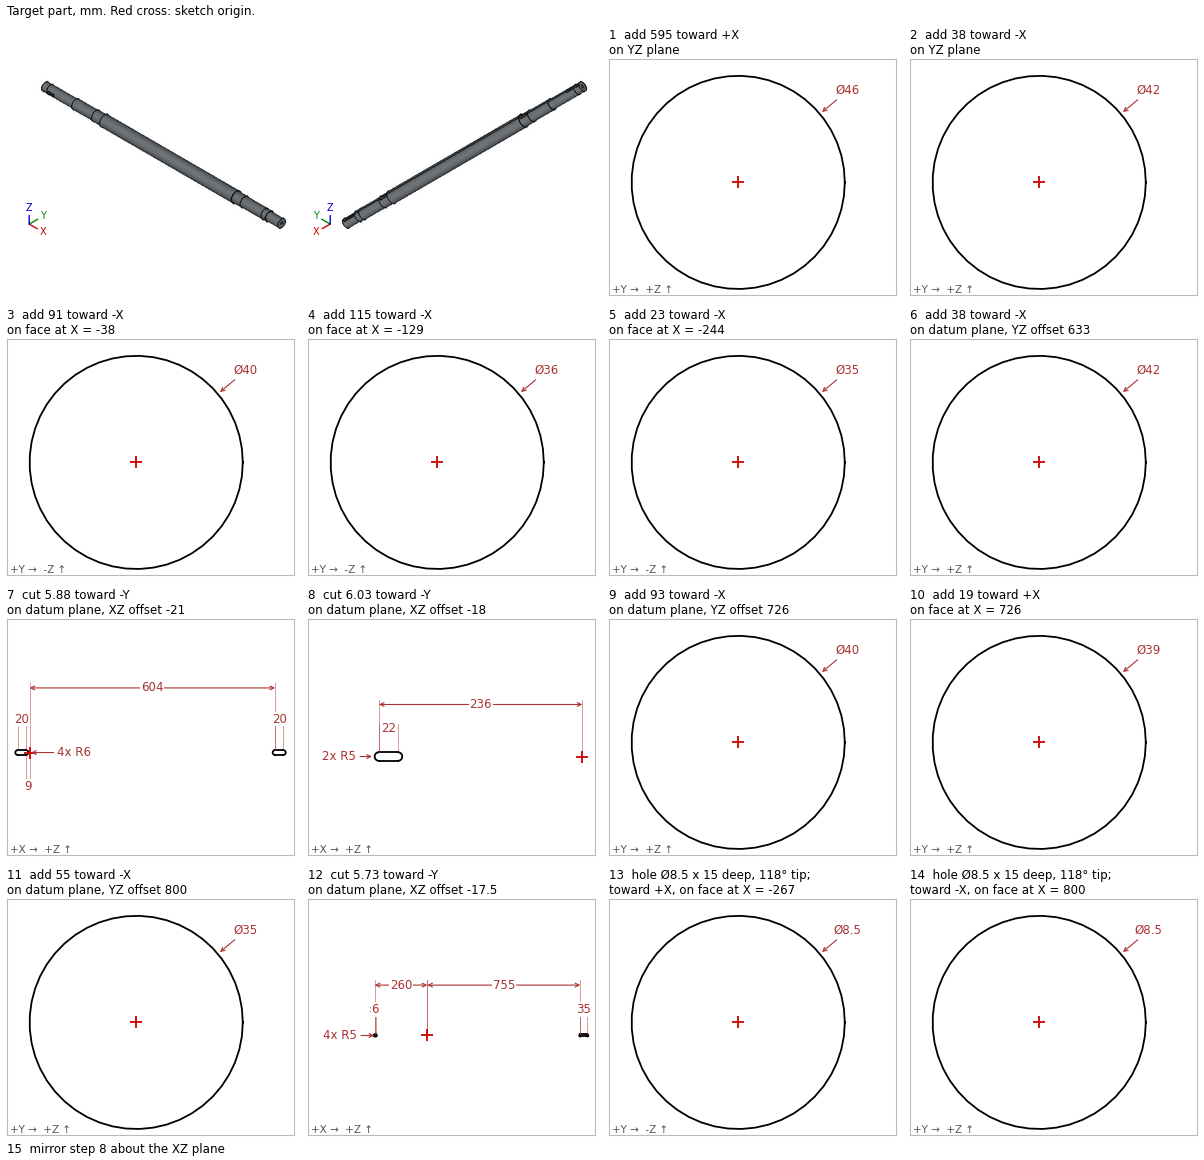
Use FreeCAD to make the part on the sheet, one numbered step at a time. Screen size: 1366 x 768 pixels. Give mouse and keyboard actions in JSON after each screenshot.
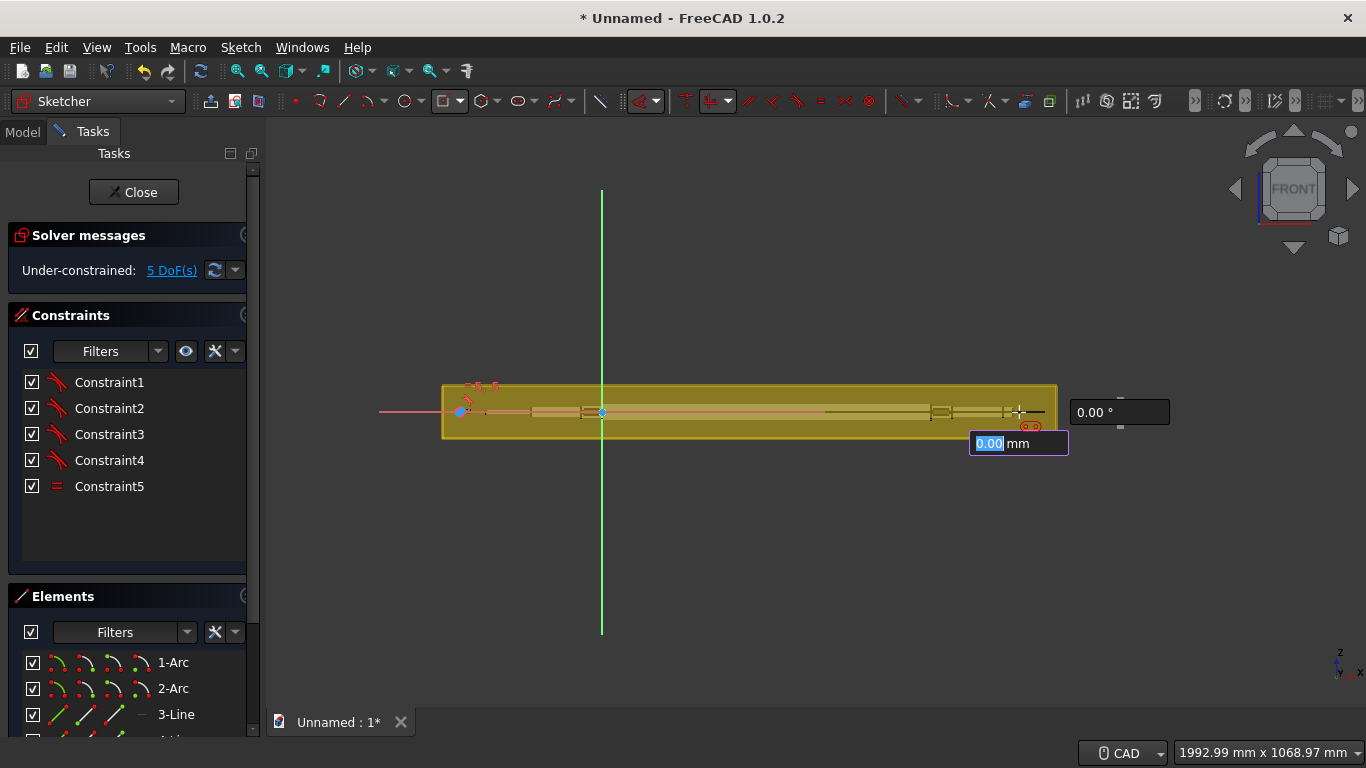
{"action": "left_click", "coordinate": [1038, 403]}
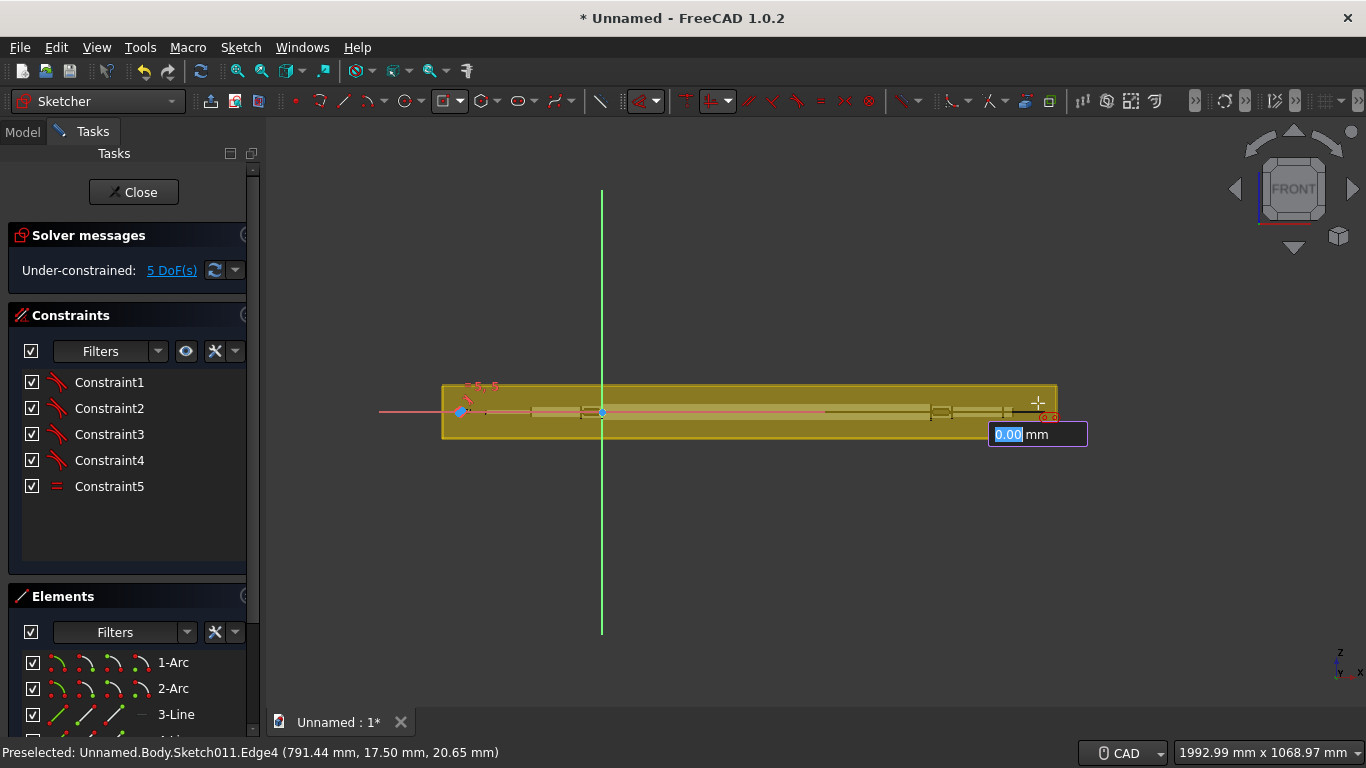
{"action": "scroll", "coordinate": [1029, 409], "scroll_direction": "up", "scroll_amount": 9}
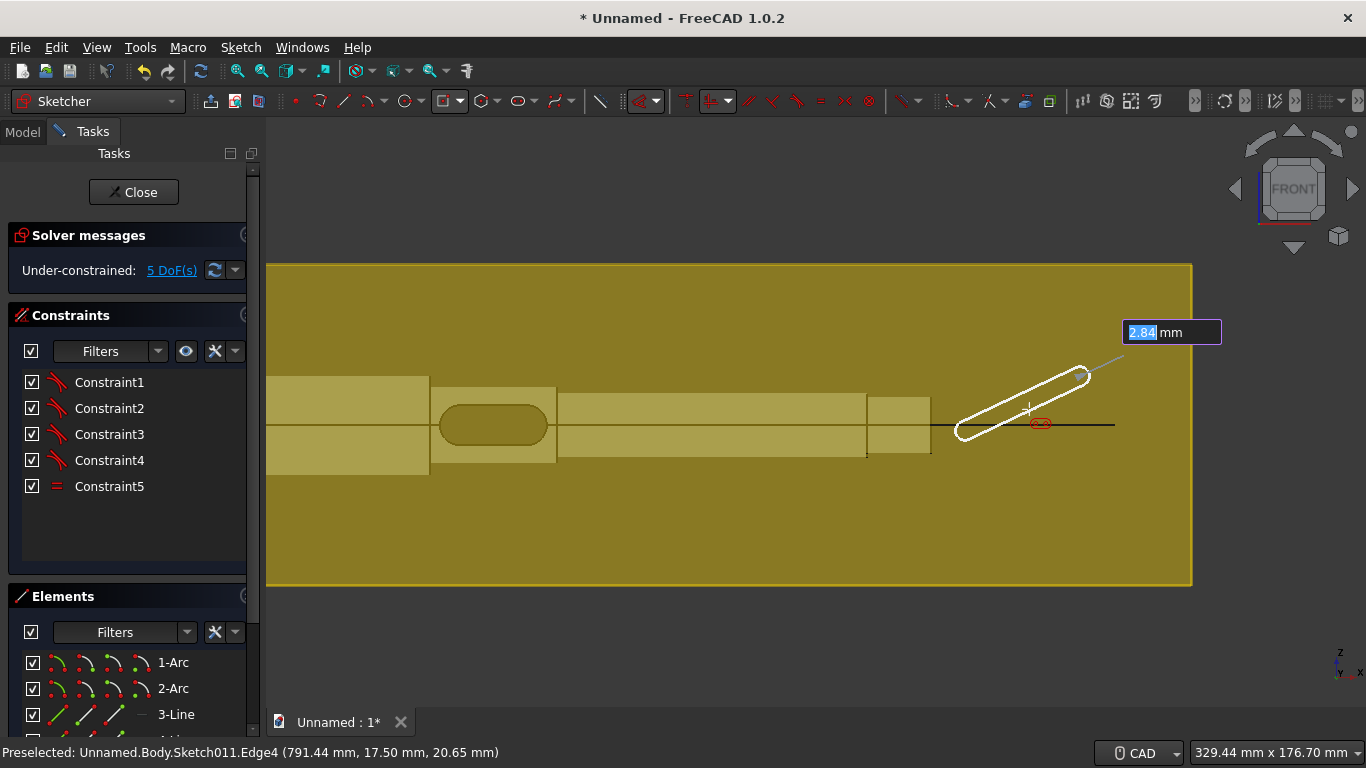
{"action": "left_click", "coordinate": [1023, 409]}
{"action": "key", "text": "Escape"}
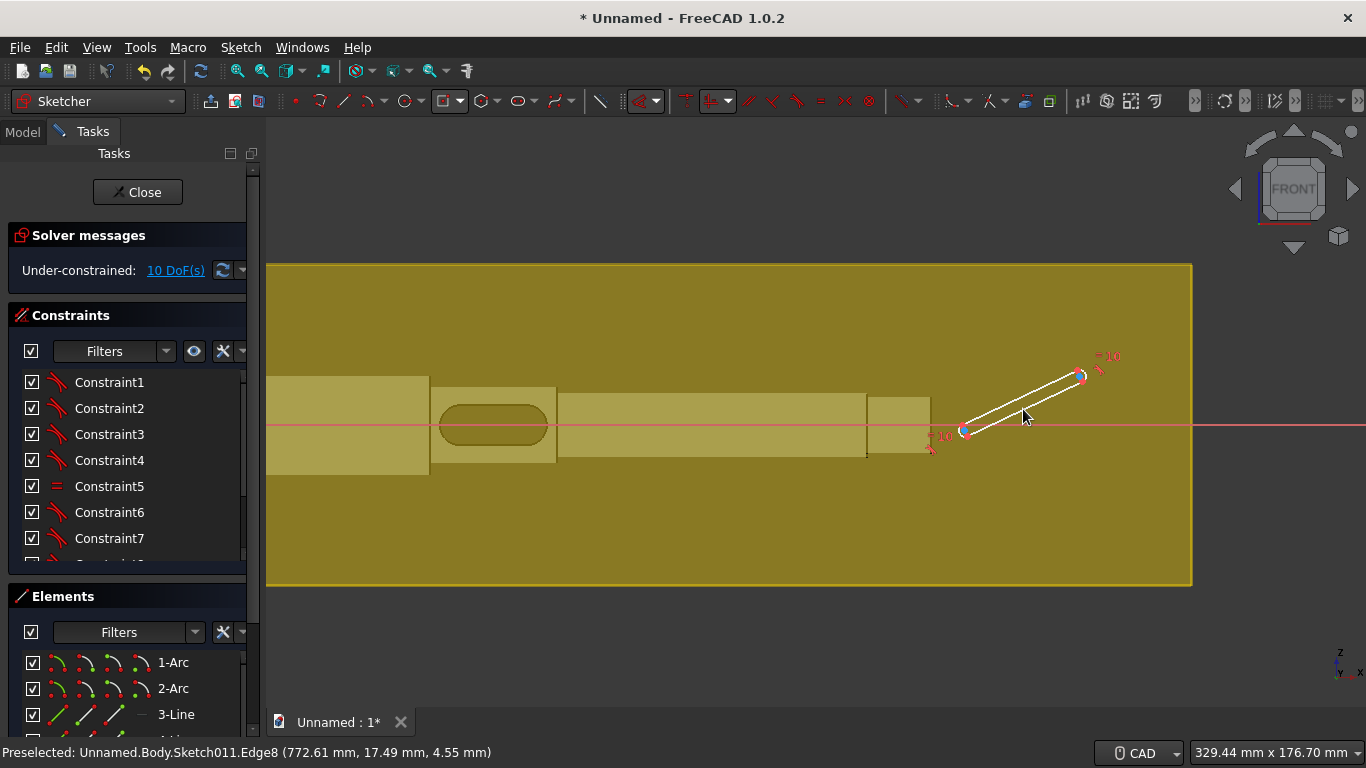
{"action": "scroll", "coordinate": [1029, 409], "scroll_direction": "down", "scroll_amount": 9}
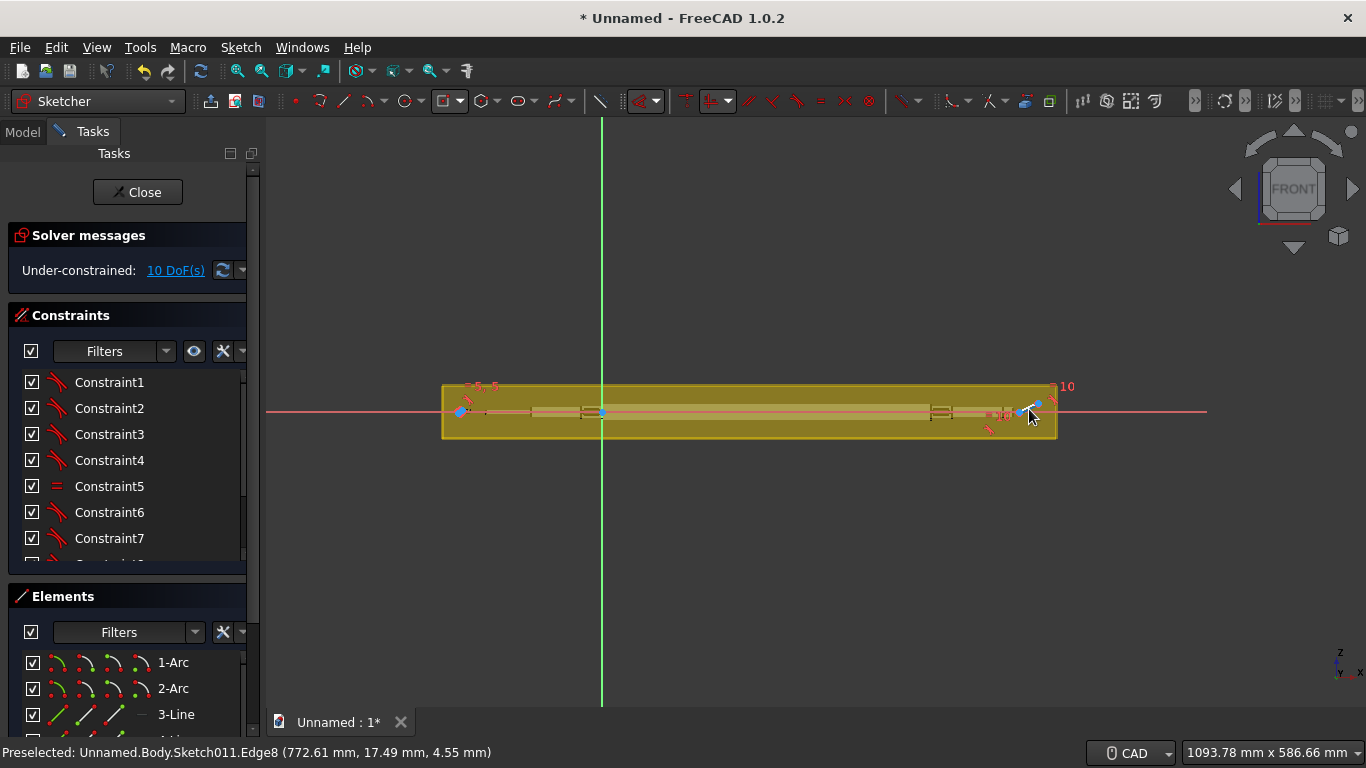
{"action": "scroll", "coordinate": [460, 410], "scroll_direction": "up", "scroll_amount": 11}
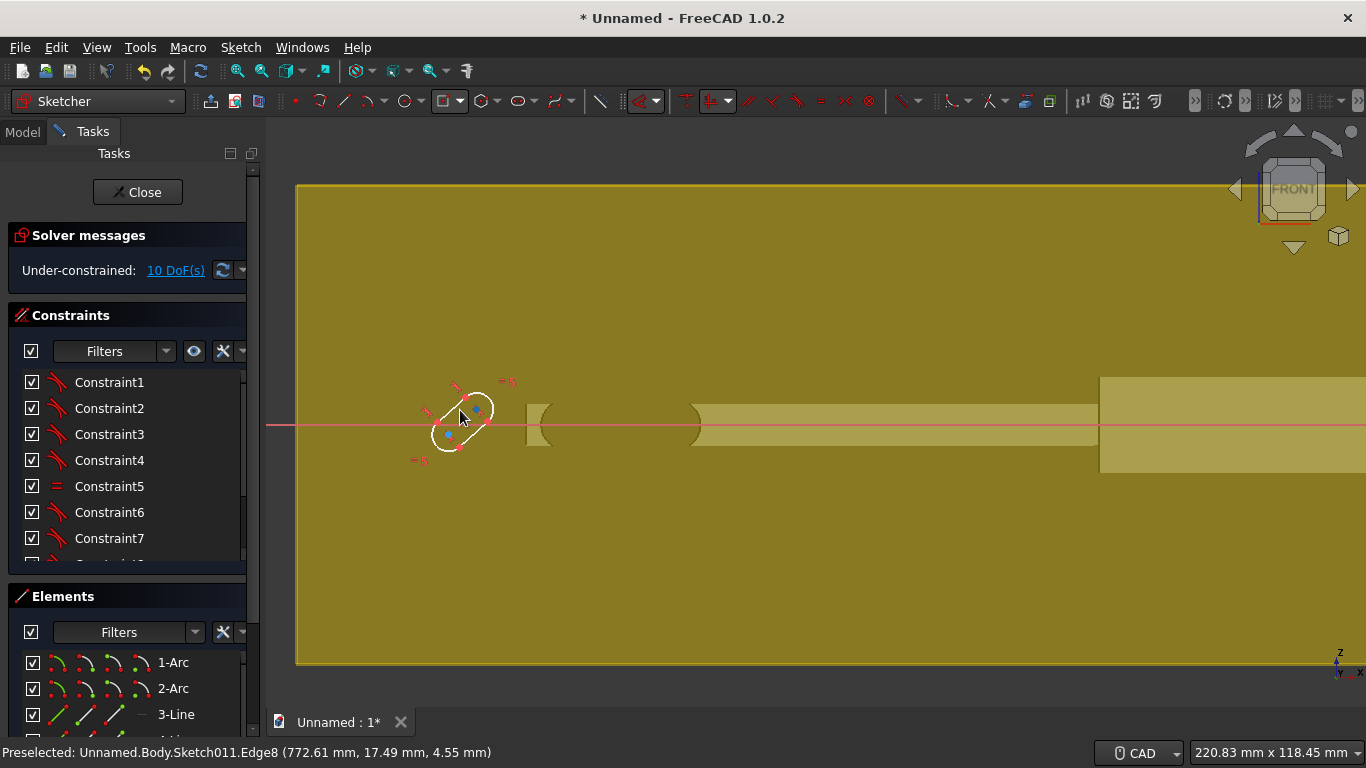
{"action": "left_click", "coordinate": [455, 407]}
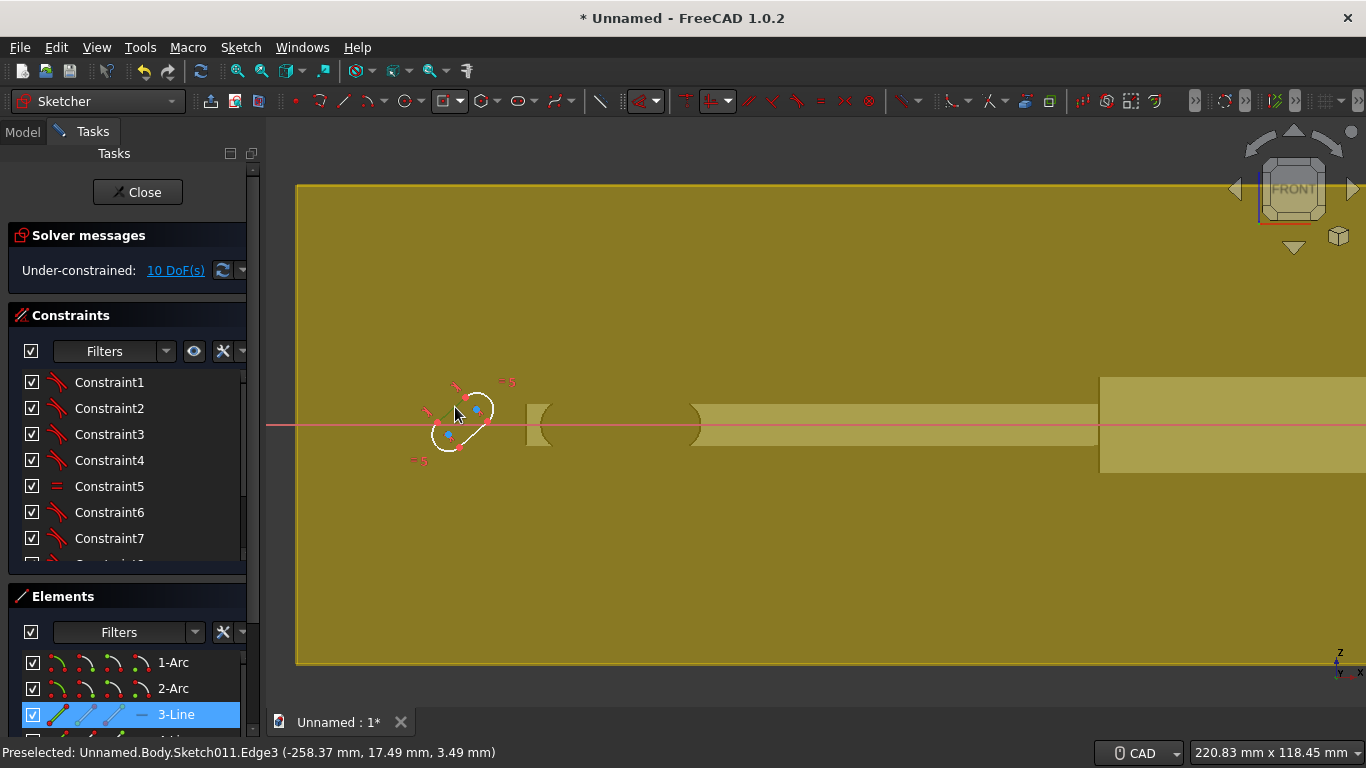
{"action": "key", "text": "h"}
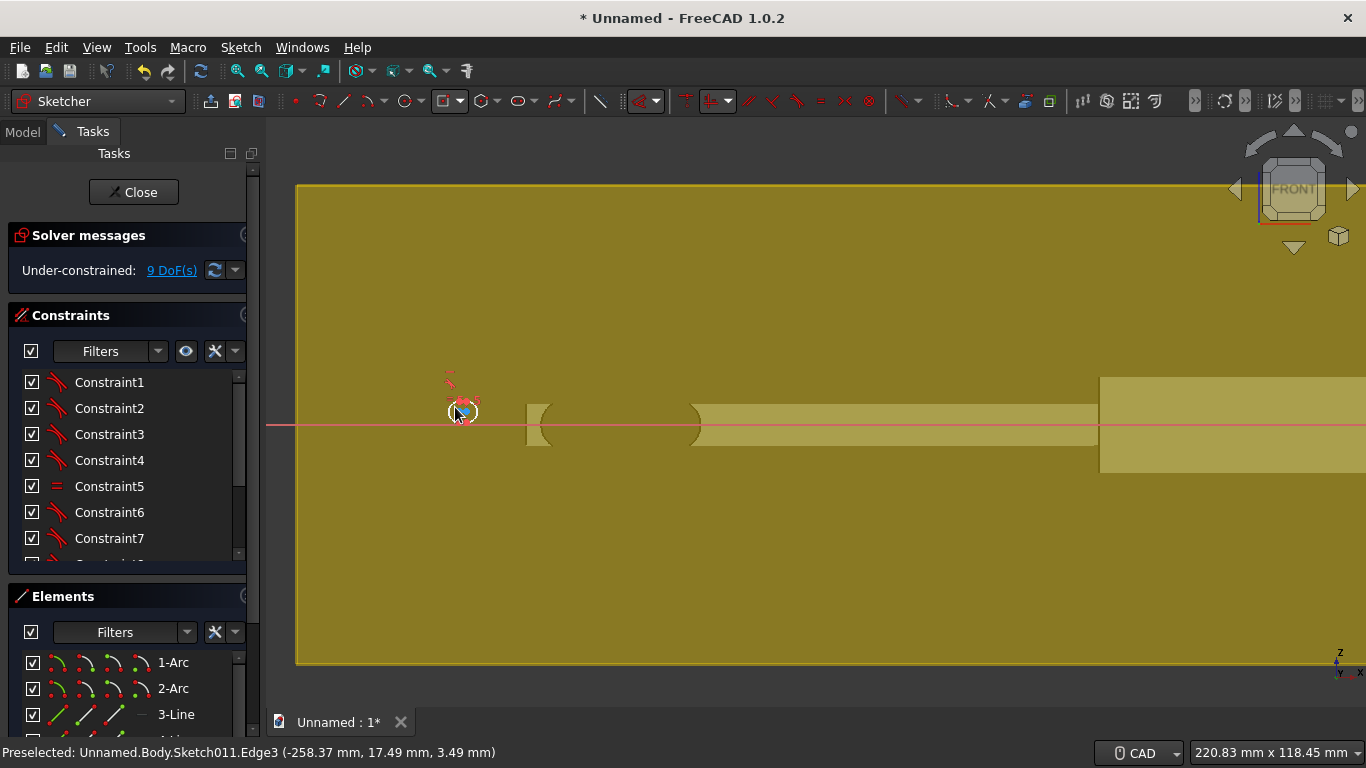
{"action": "scroll", "coordinate": [459, 410], "scroll_direction": "down", "scroll_amount": 11}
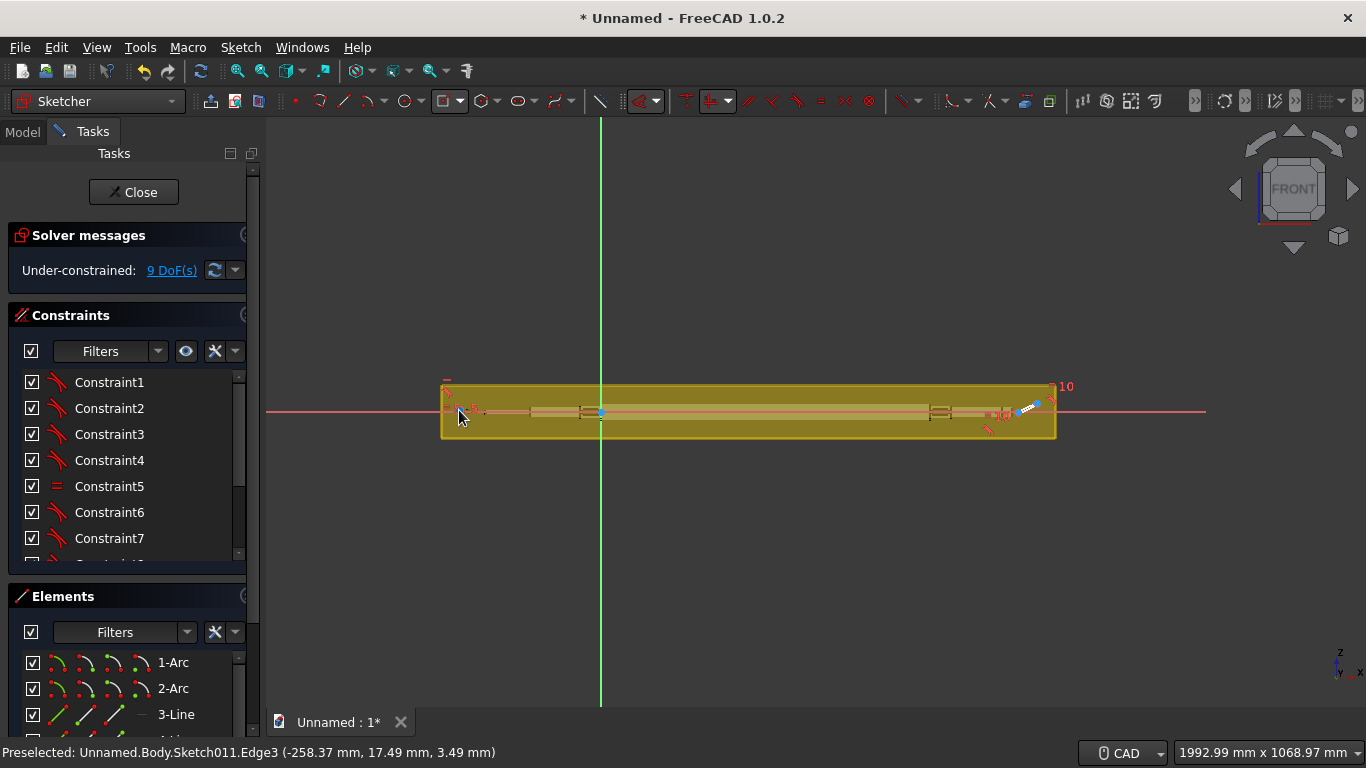
{"action": "scroll", "coordinate": [1023, 409], "scroll_direction": "up", "scroll_amount": 10}